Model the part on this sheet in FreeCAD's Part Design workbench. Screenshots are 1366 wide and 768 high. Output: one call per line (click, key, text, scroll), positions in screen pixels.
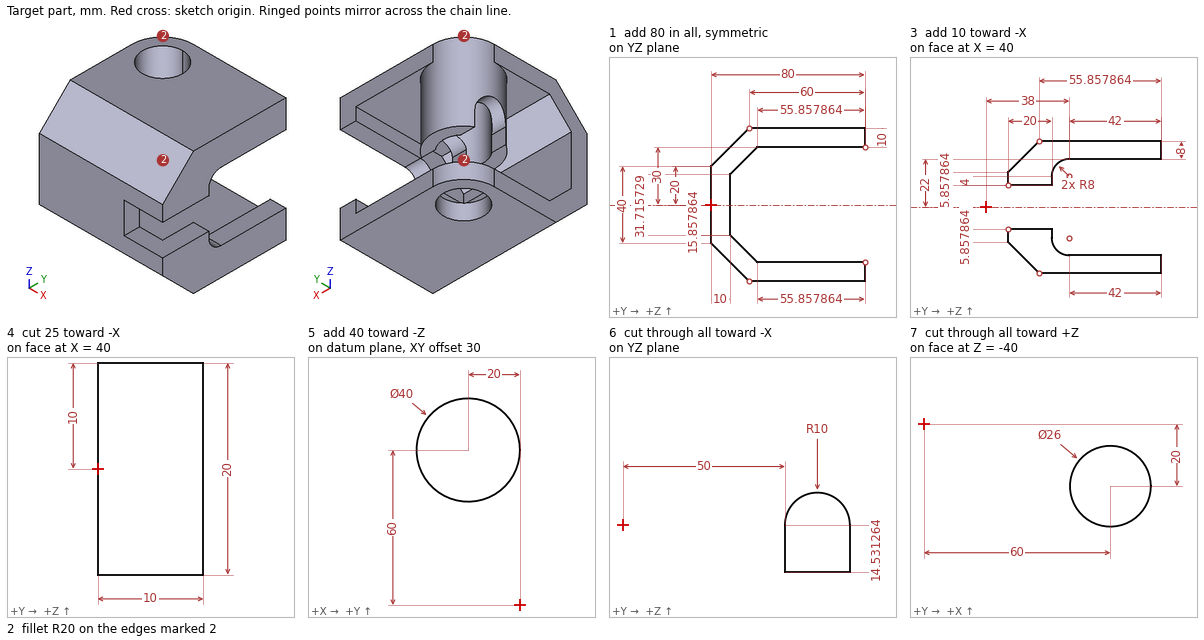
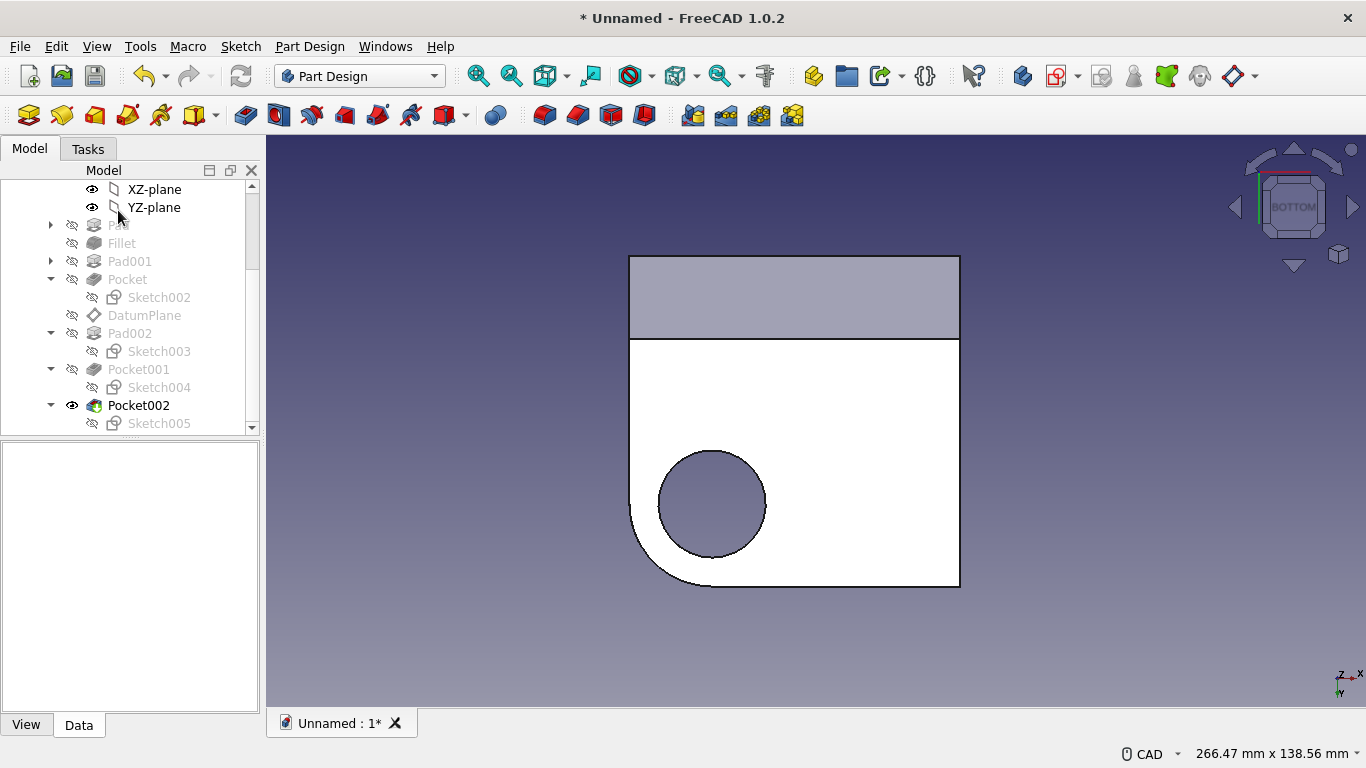
key(0)